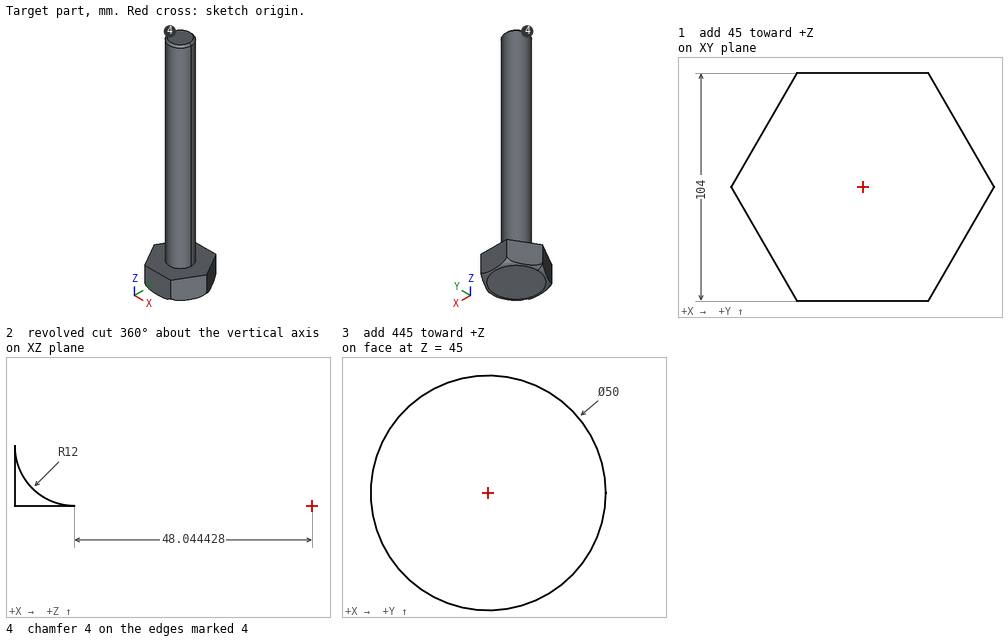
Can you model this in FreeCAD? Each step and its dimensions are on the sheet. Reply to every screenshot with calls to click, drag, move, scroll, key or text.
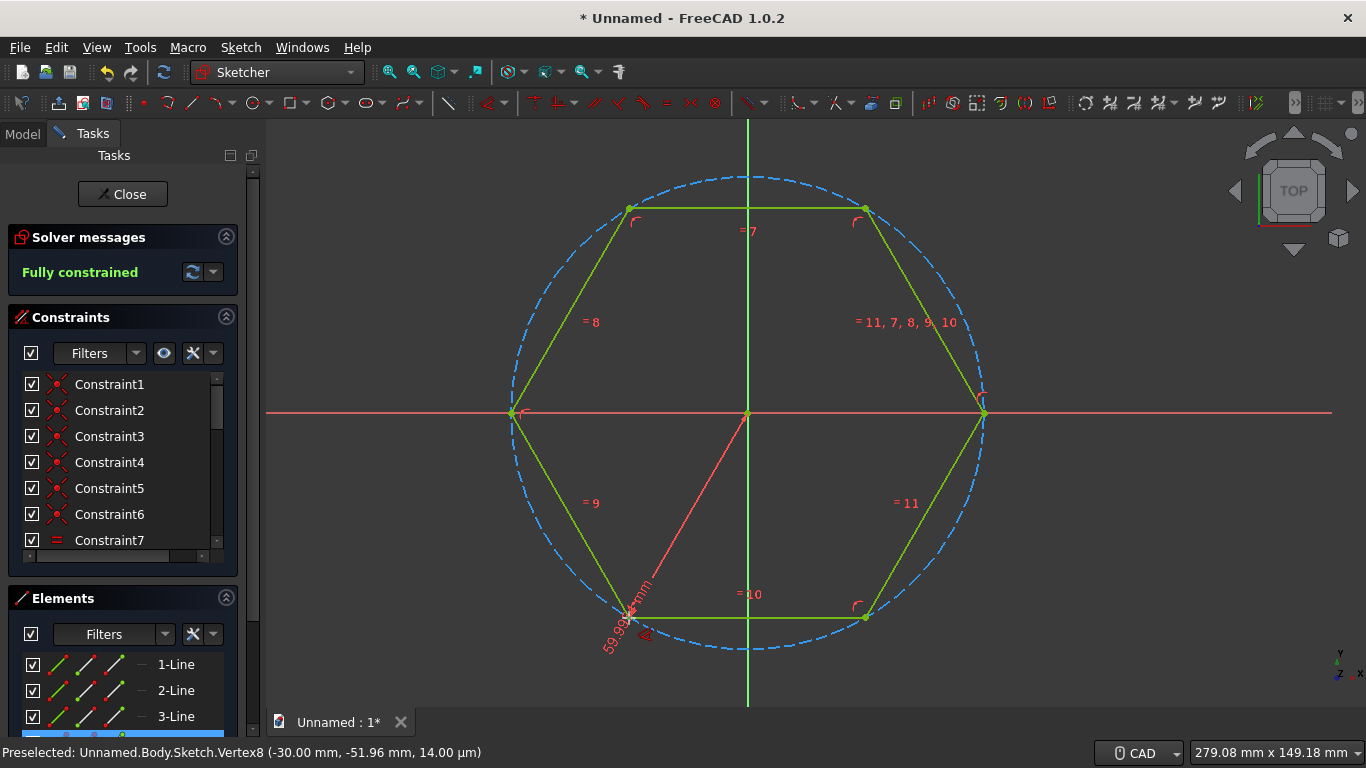
click(866, 208)
click(900, 319)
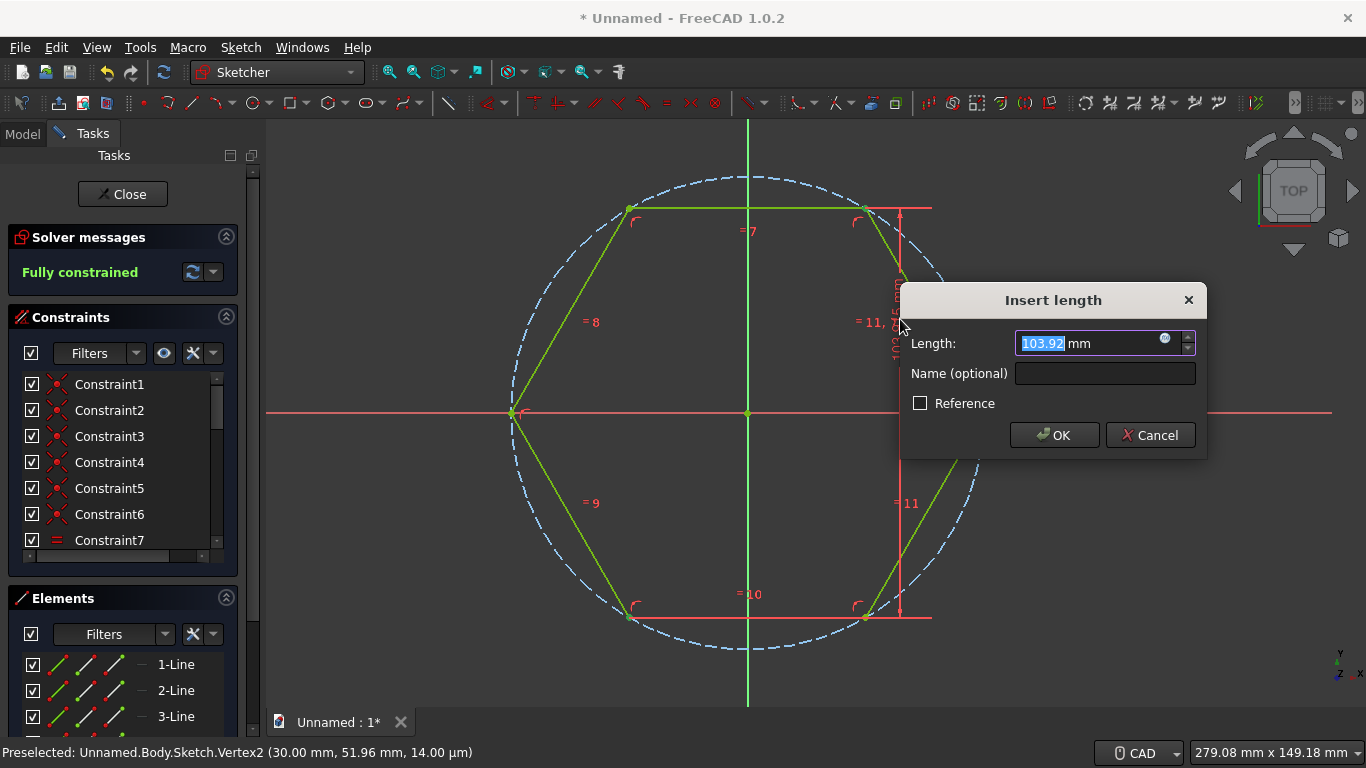
text(104)
key(Return)
key(Escape)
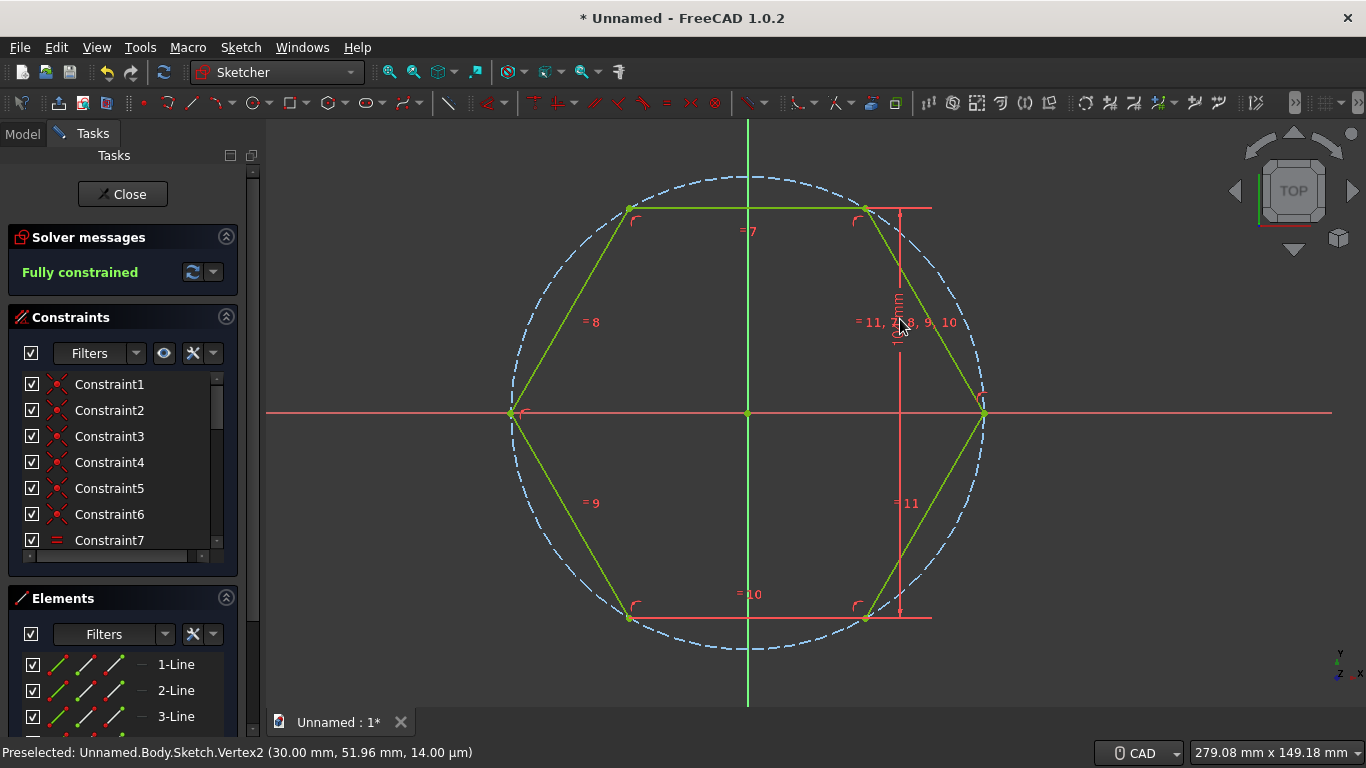
click(123, 194)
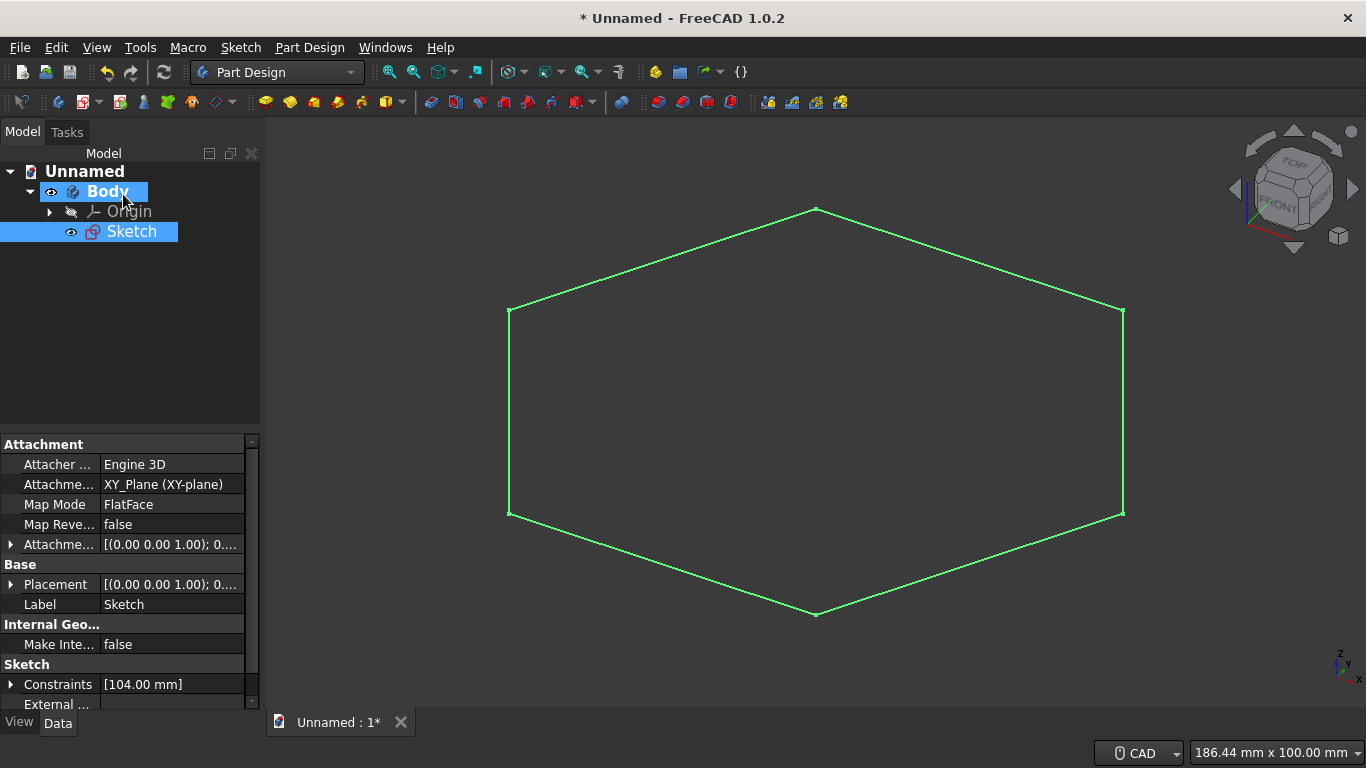
click(266, 102)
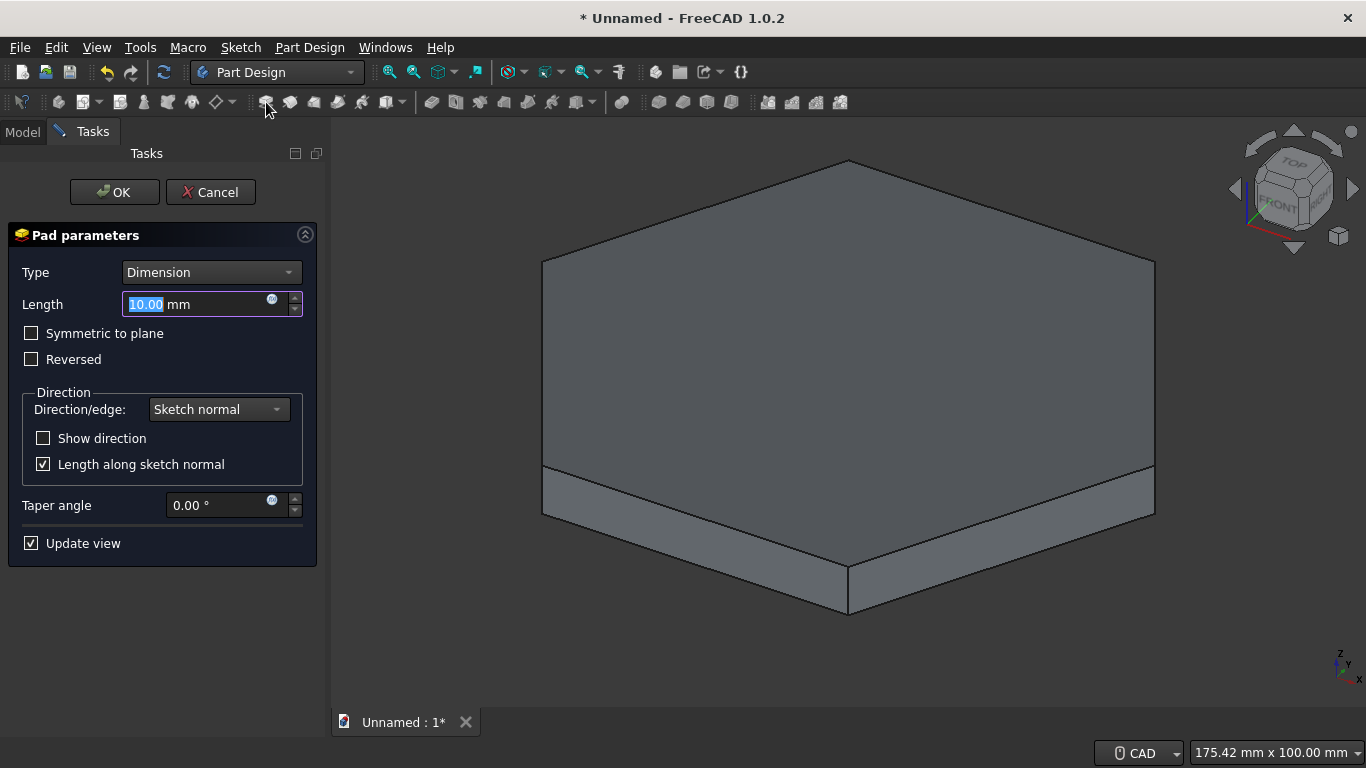
text(45)
key(Tab)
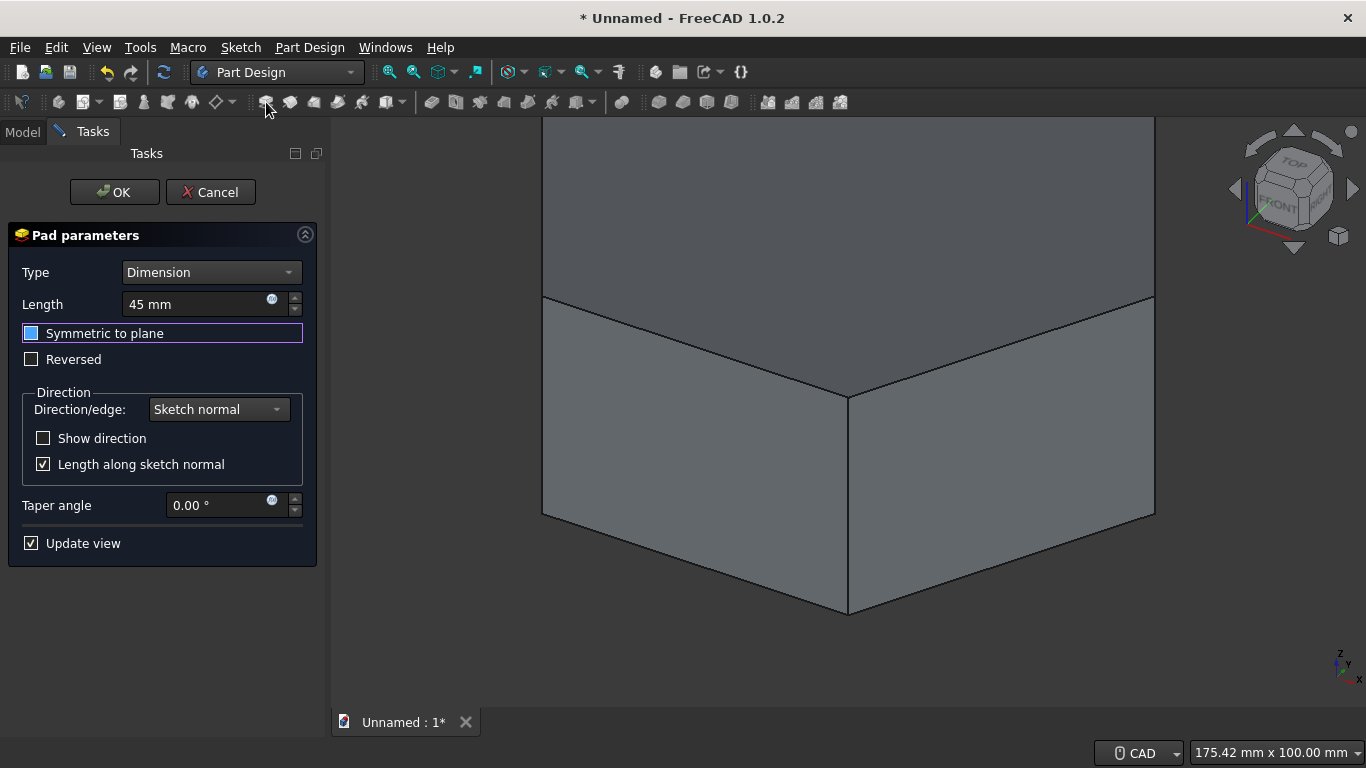
click(115, 192)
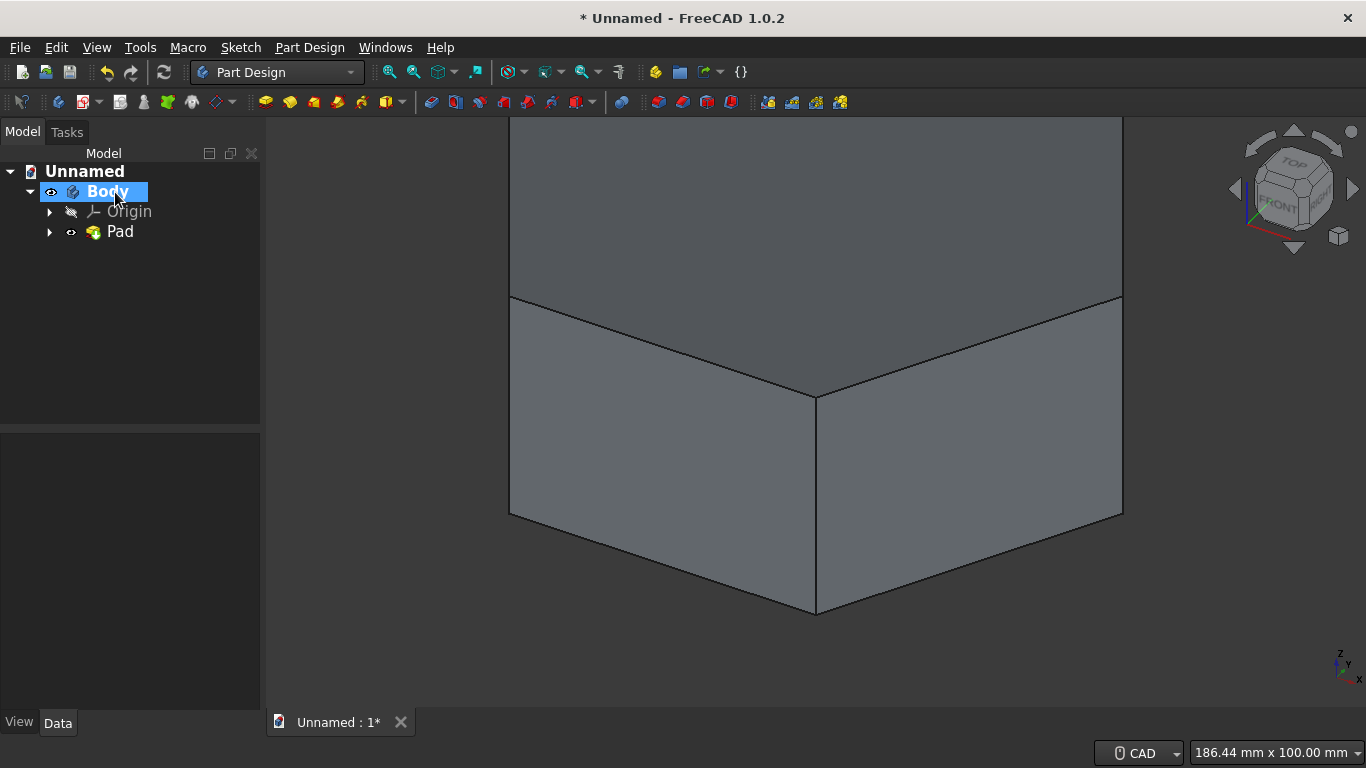
click(390, 72)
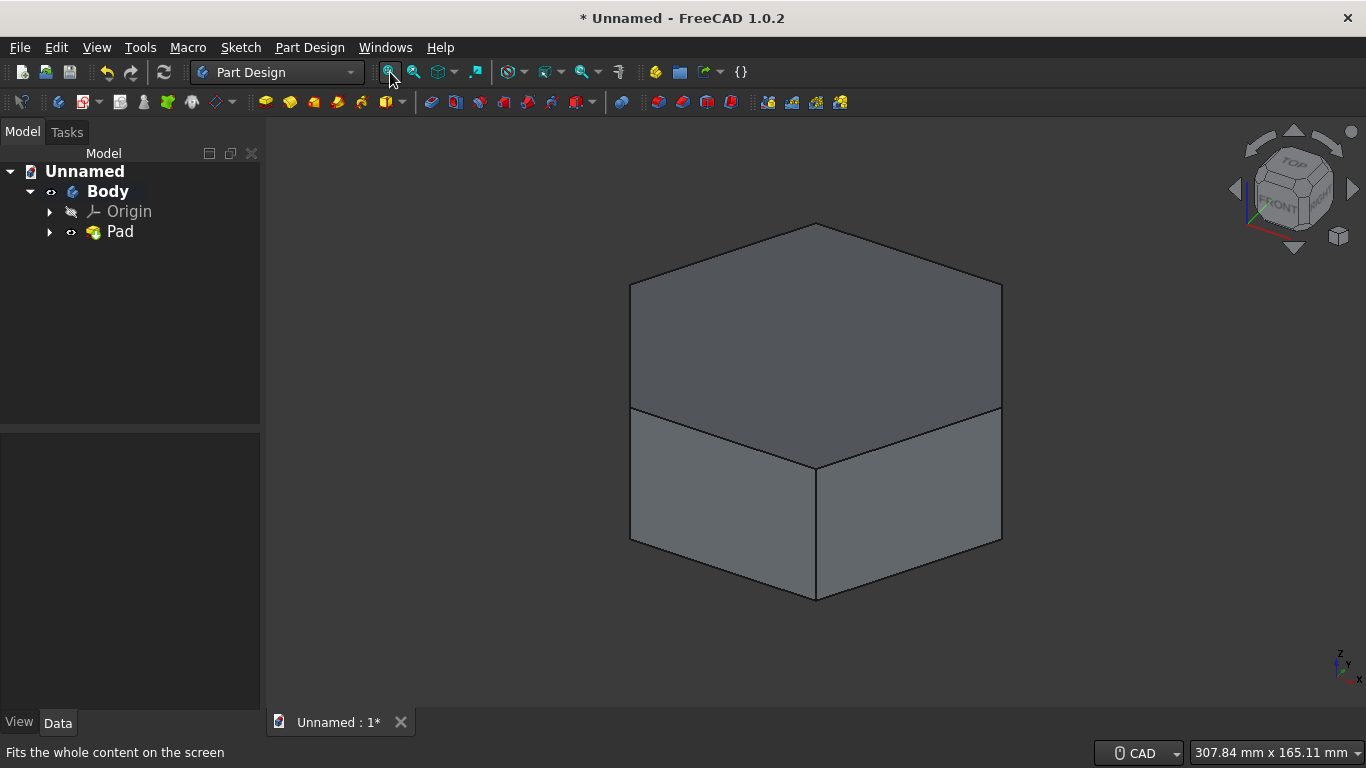
click(84, 102)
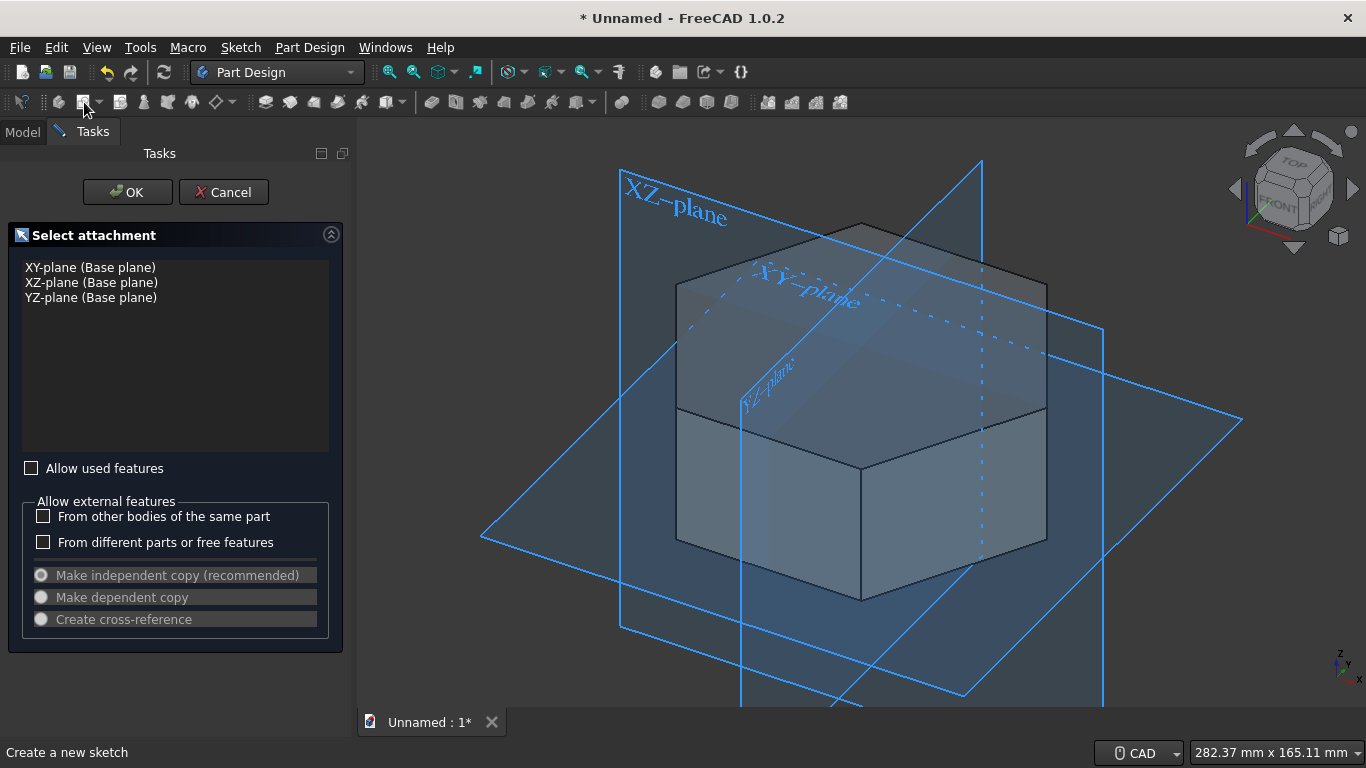
click(82, 282)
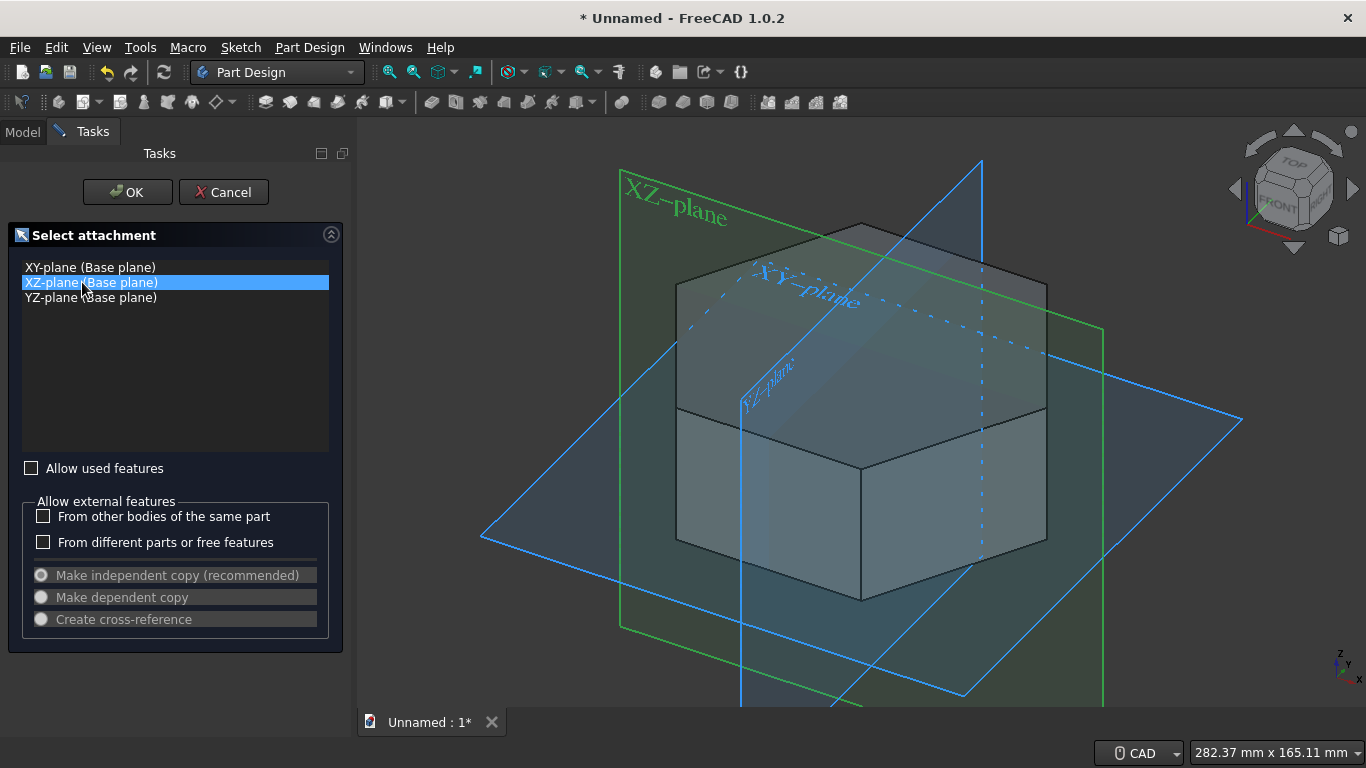
click(128, 192)